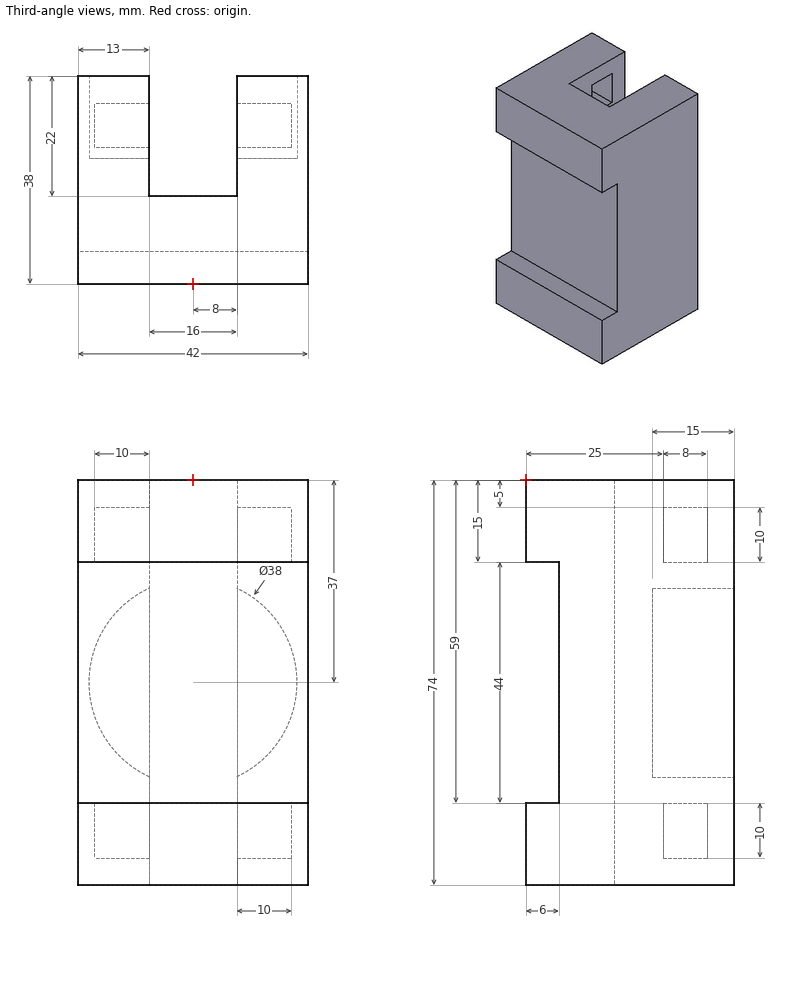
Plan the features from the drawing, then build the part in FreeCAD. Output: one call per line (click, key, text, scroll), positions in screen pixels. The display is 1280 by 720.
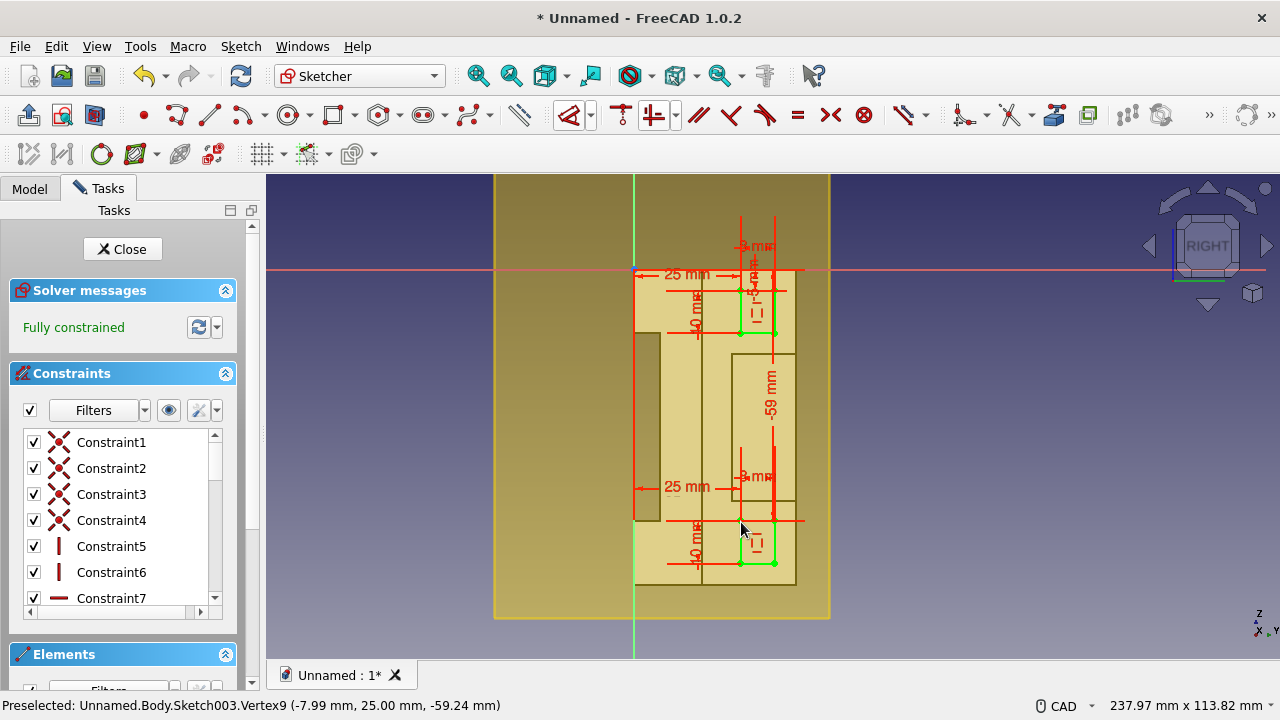
click(123, 249)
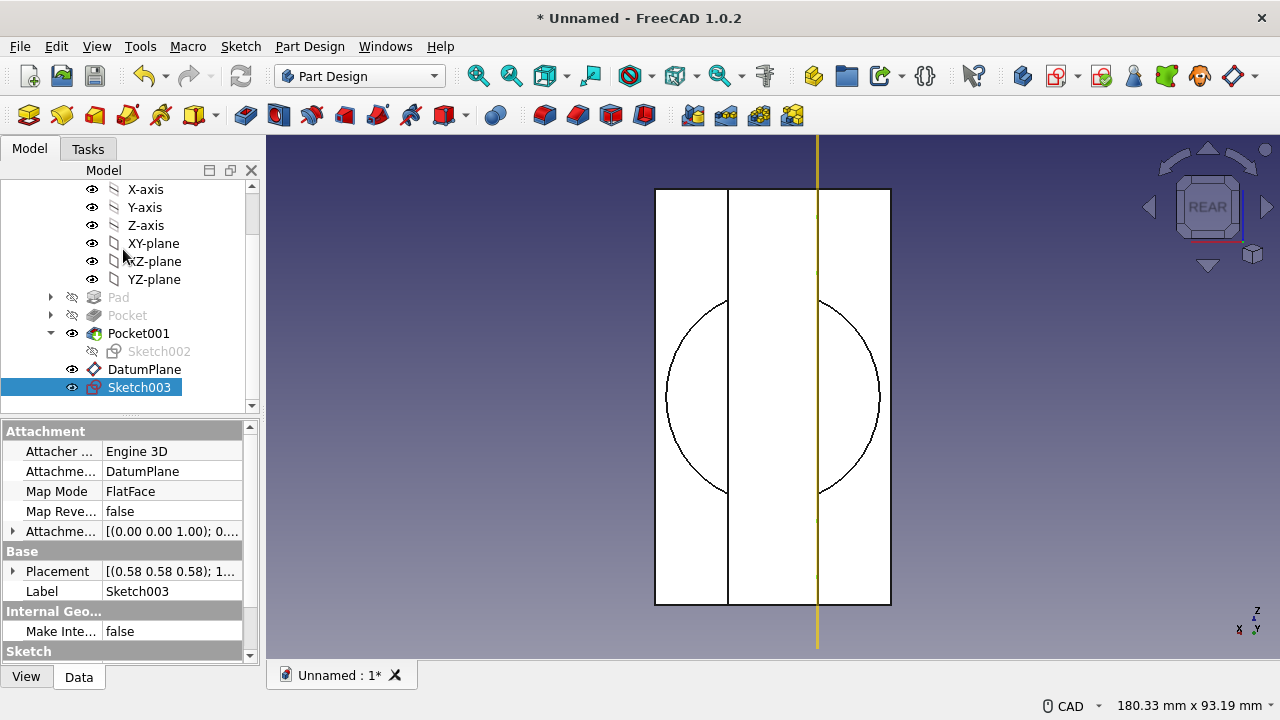
click(246, 116)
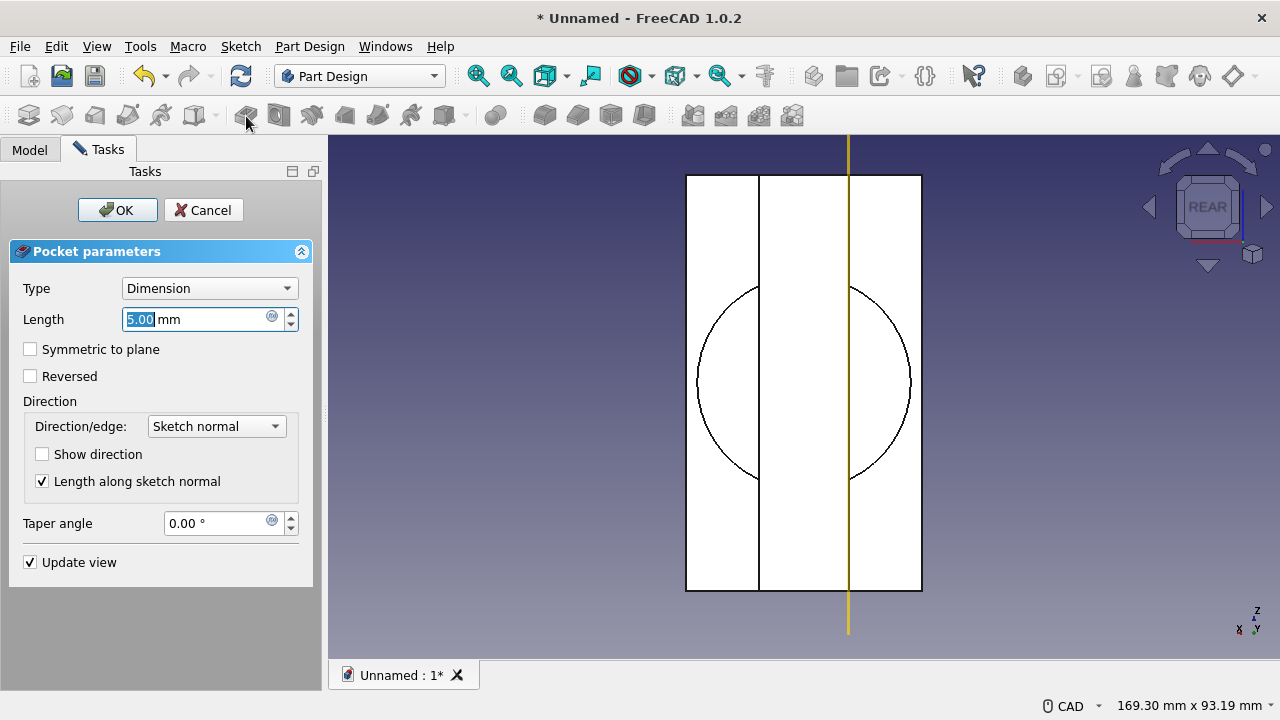
text(10)
key(Tab)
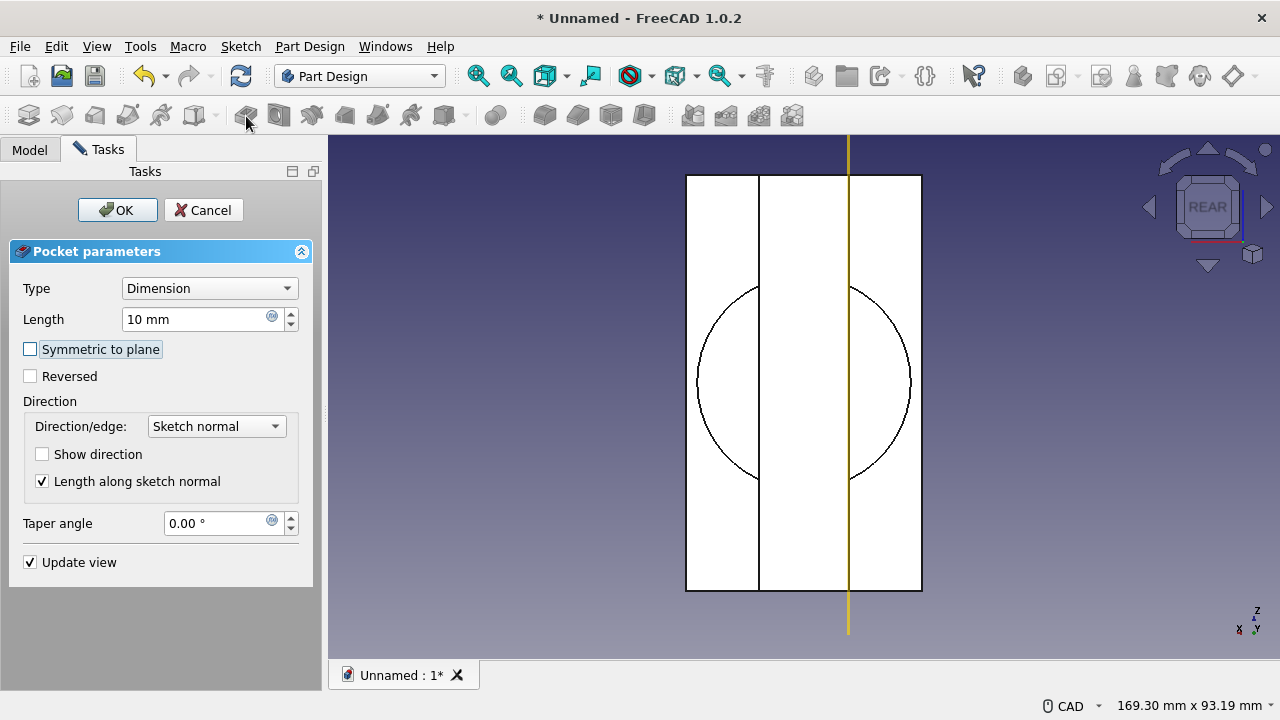
click(118, 210)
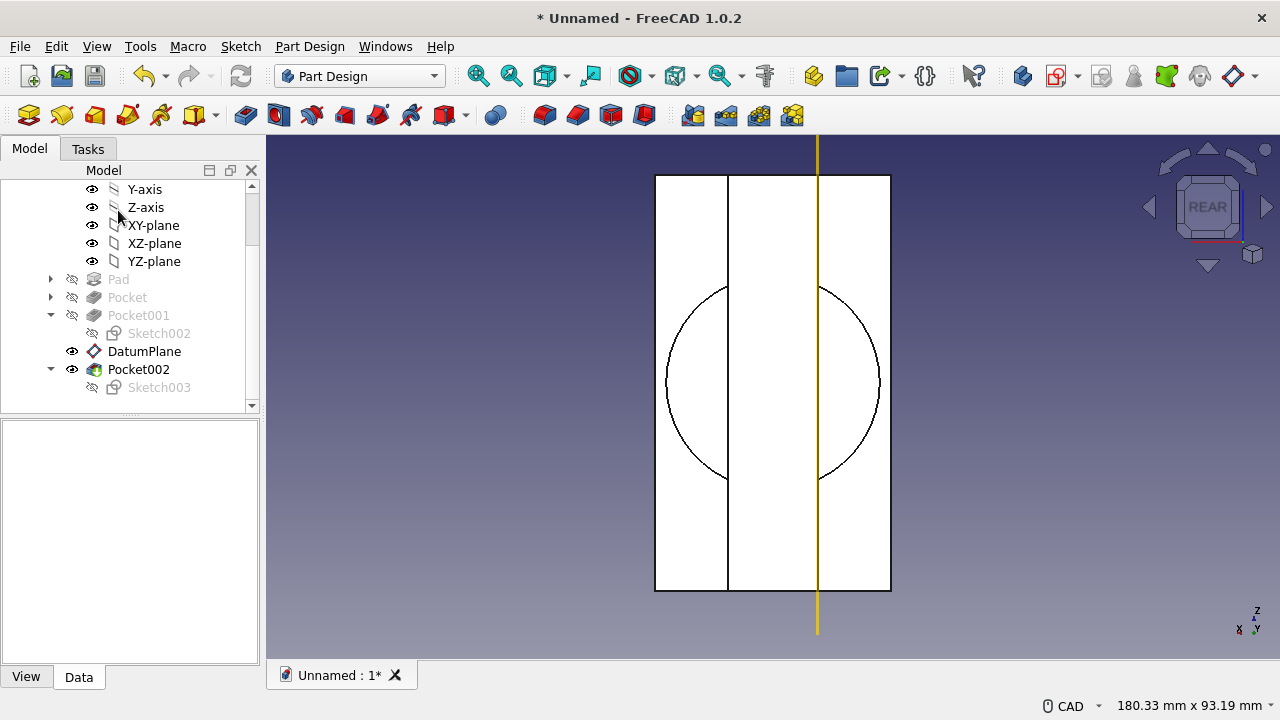
click(117, 351)
key(space)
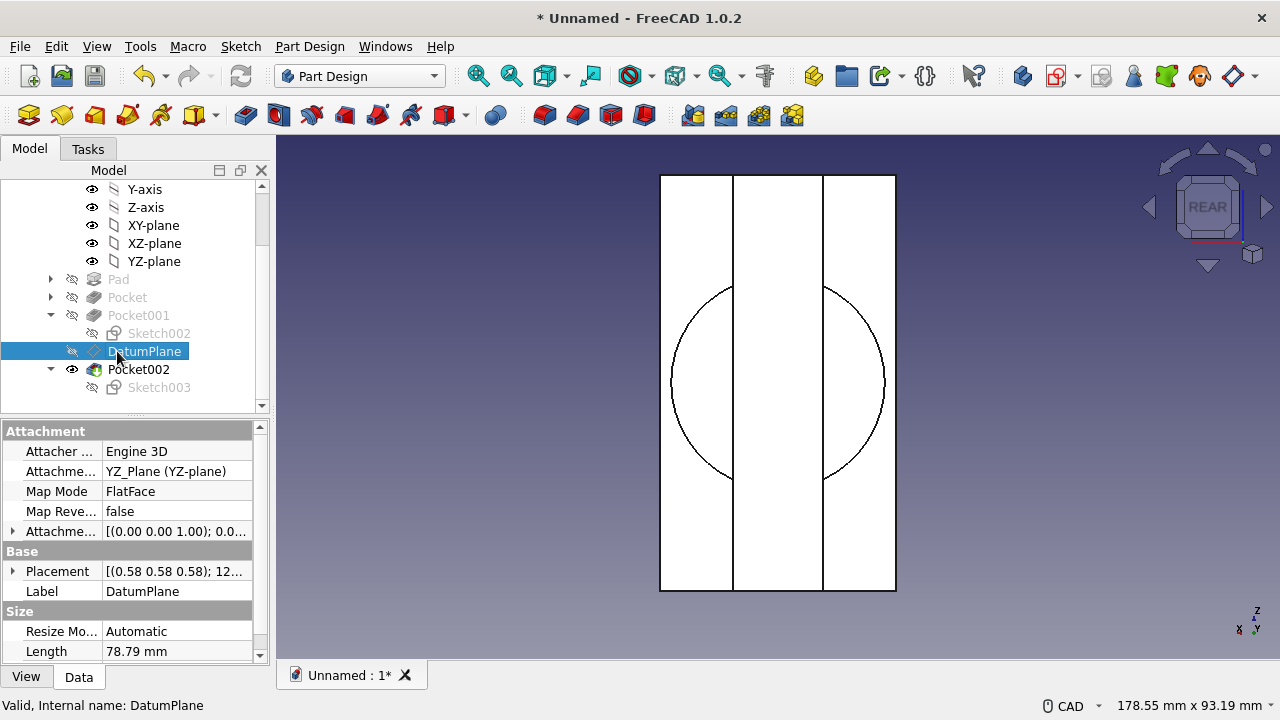
scroll(161, 293, down, 3)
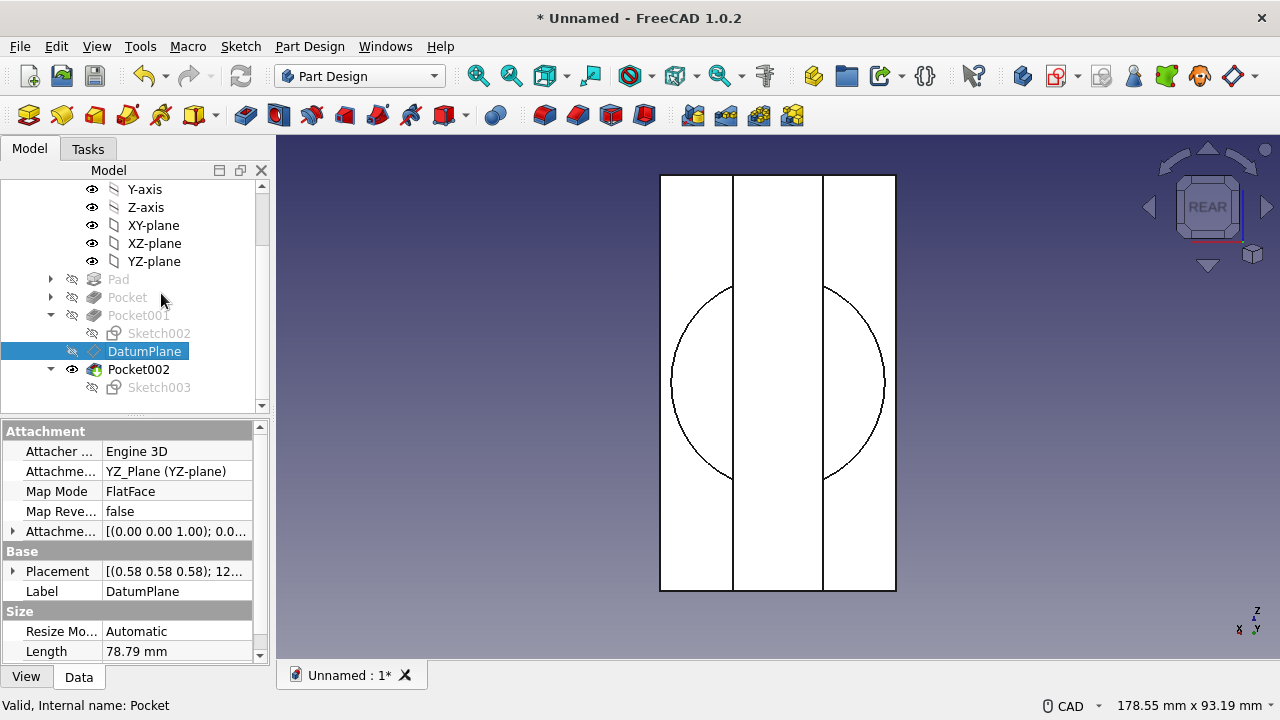
scroll(161, 293, up, 15)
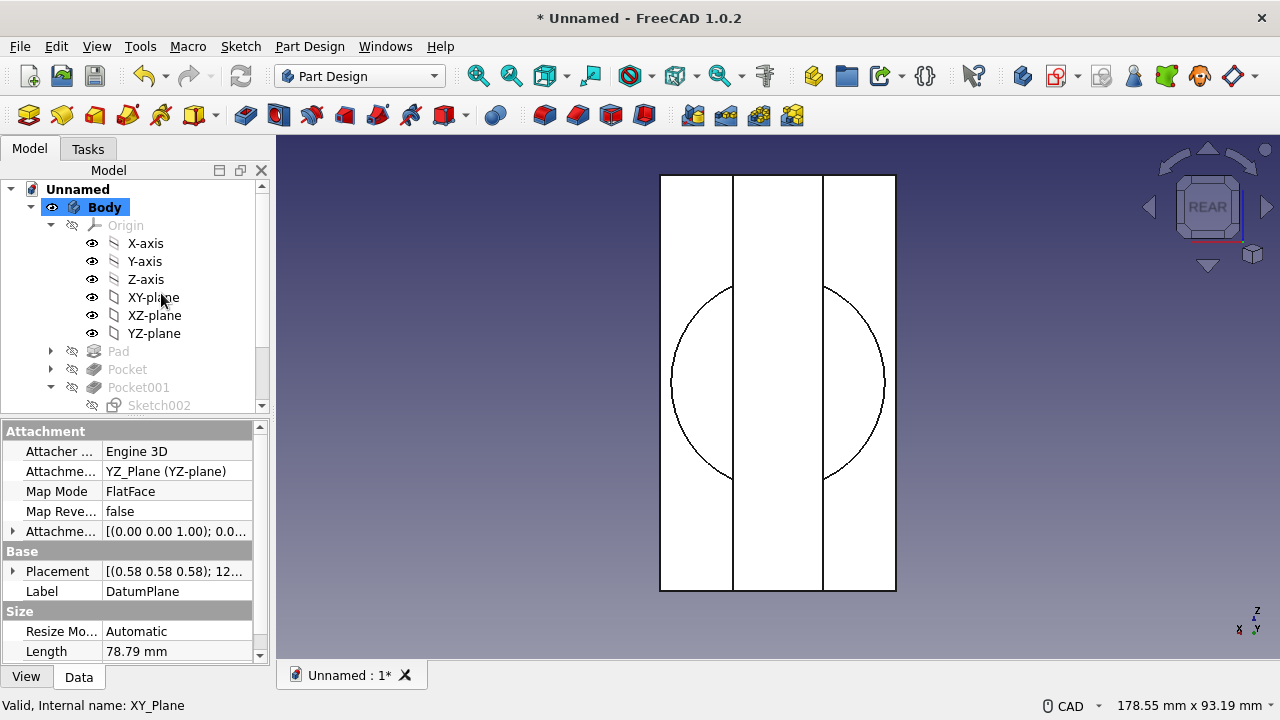
click(137, 333)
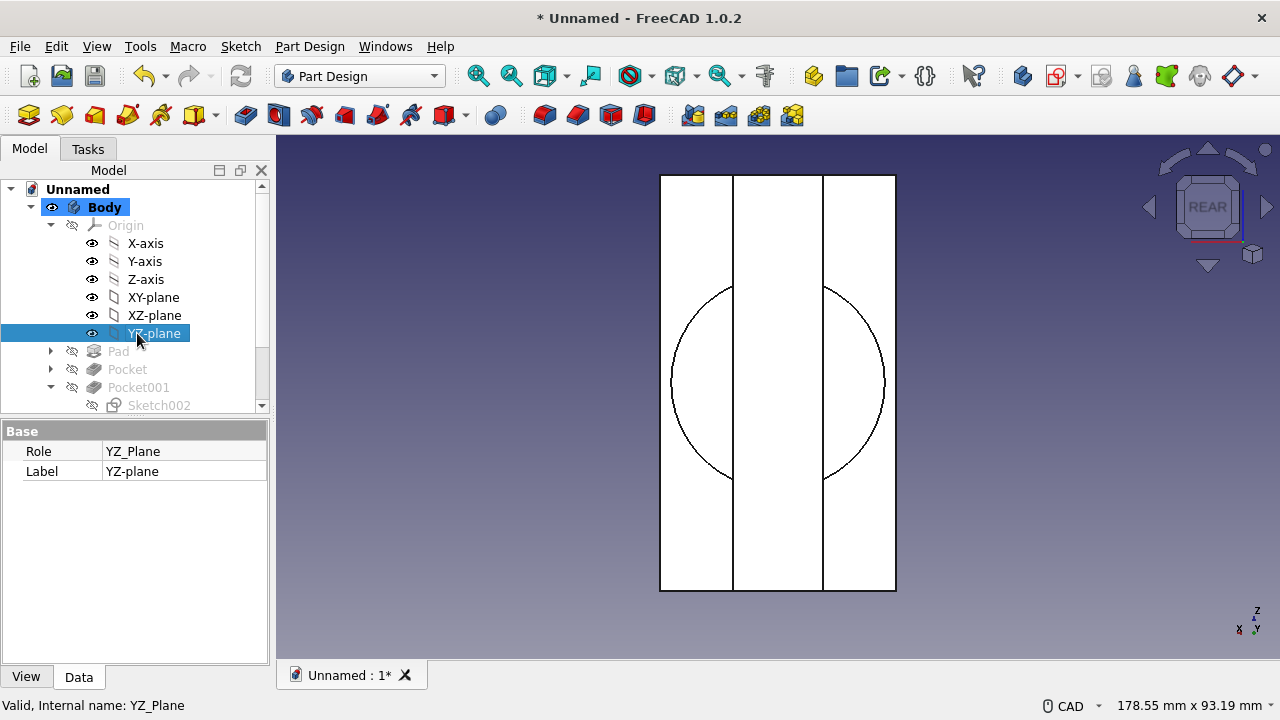
click(1232, 76)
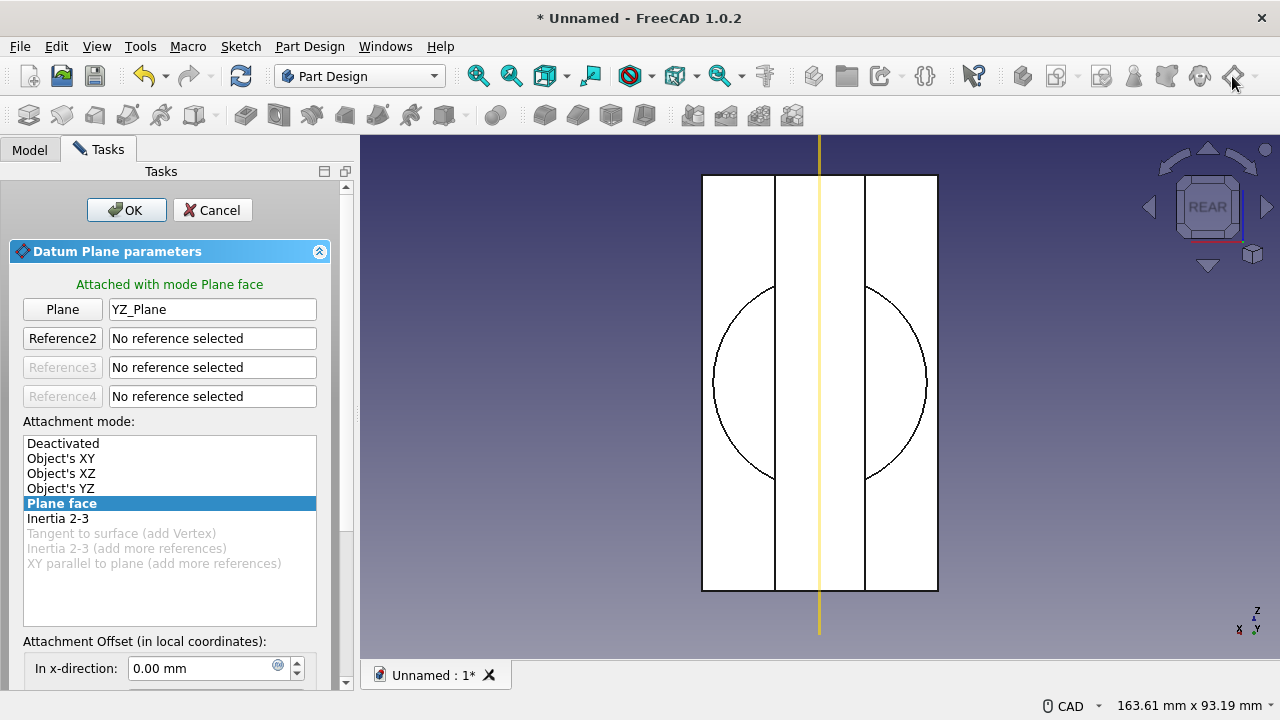
scroll(346, 436, down, 2)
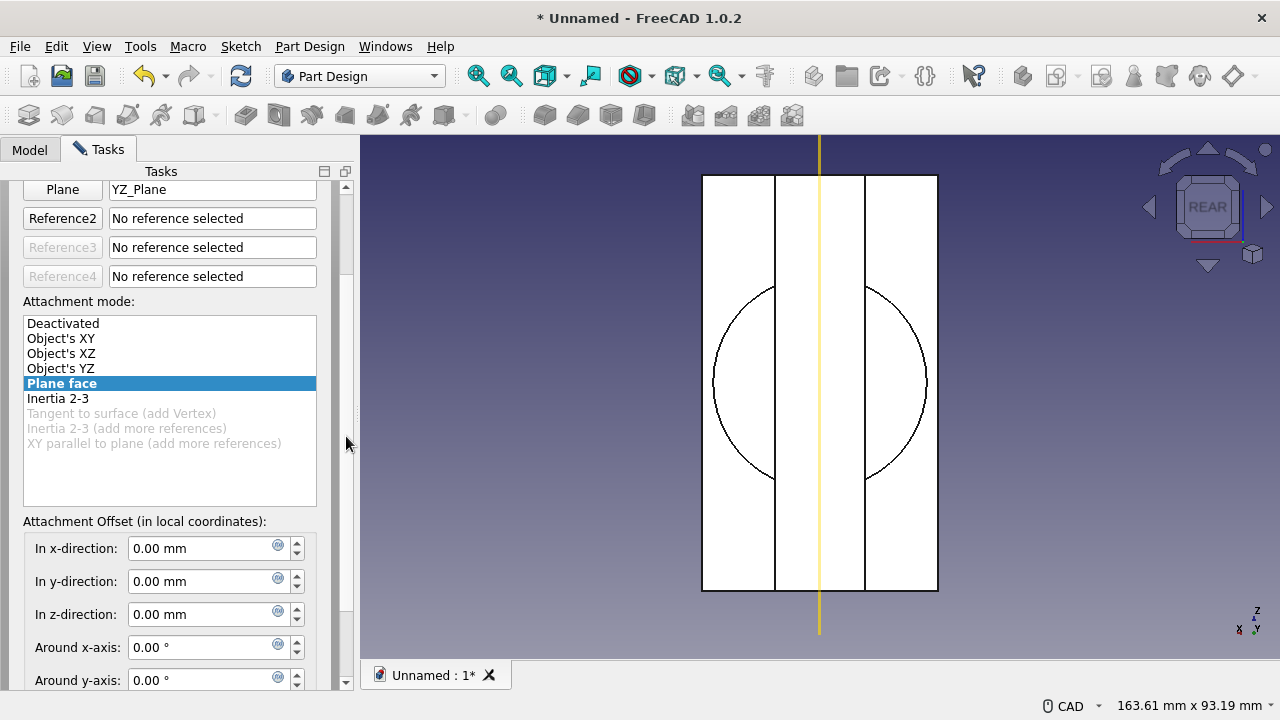
triple_click(210, 614)